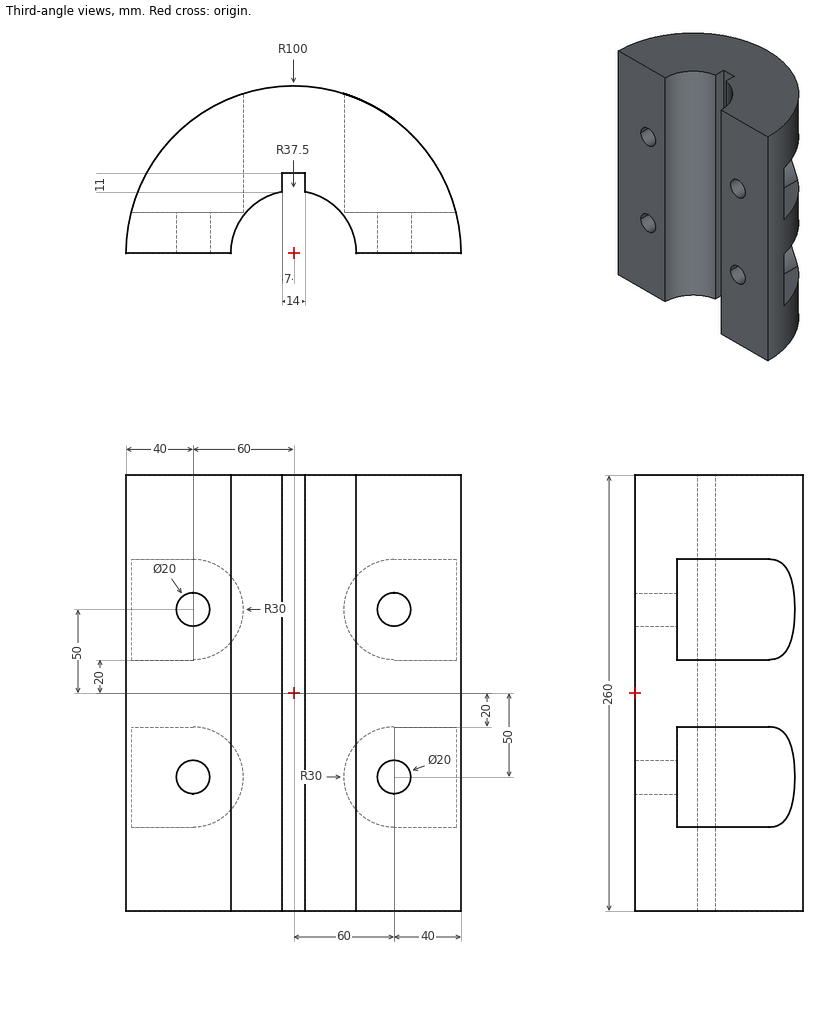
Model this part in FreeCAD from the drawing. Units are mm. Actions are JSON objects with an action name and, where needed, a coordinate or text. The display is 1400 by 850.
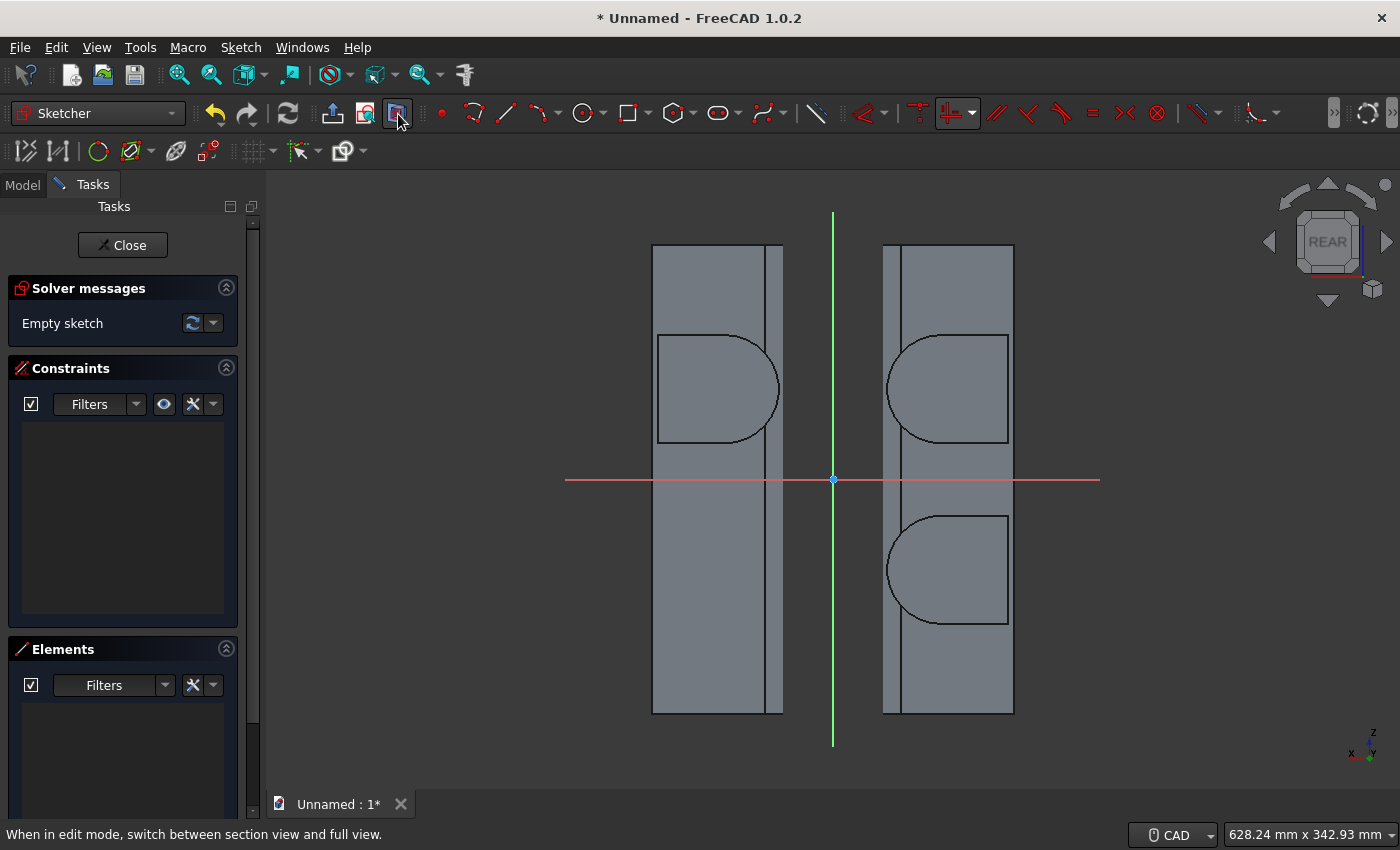
{"action": "scroll", "coordinate": [730, 594], "scroll_direction": "up", "scroll_amount": 5}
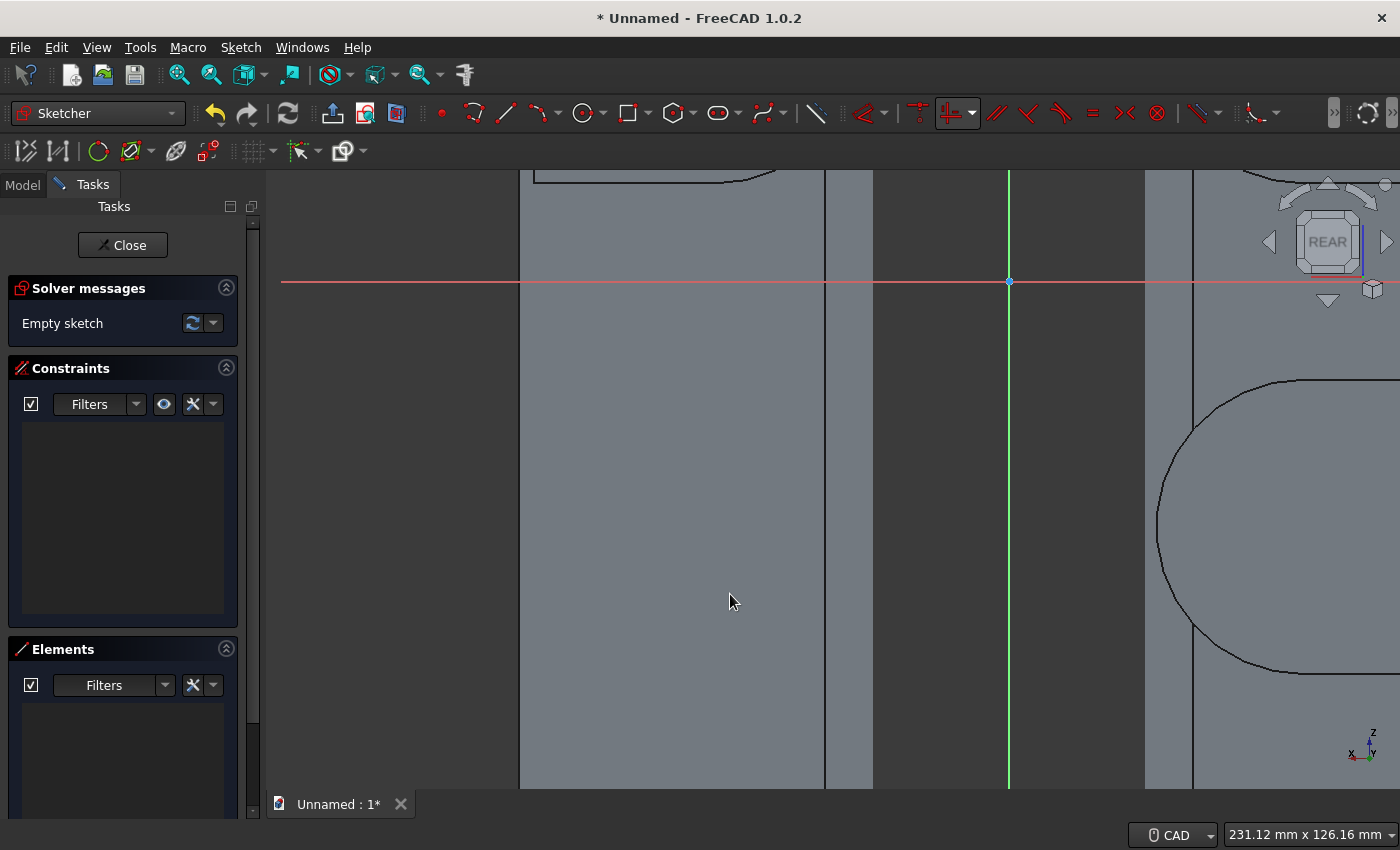
{"action": "left_click", "coordinate": [474, 114]}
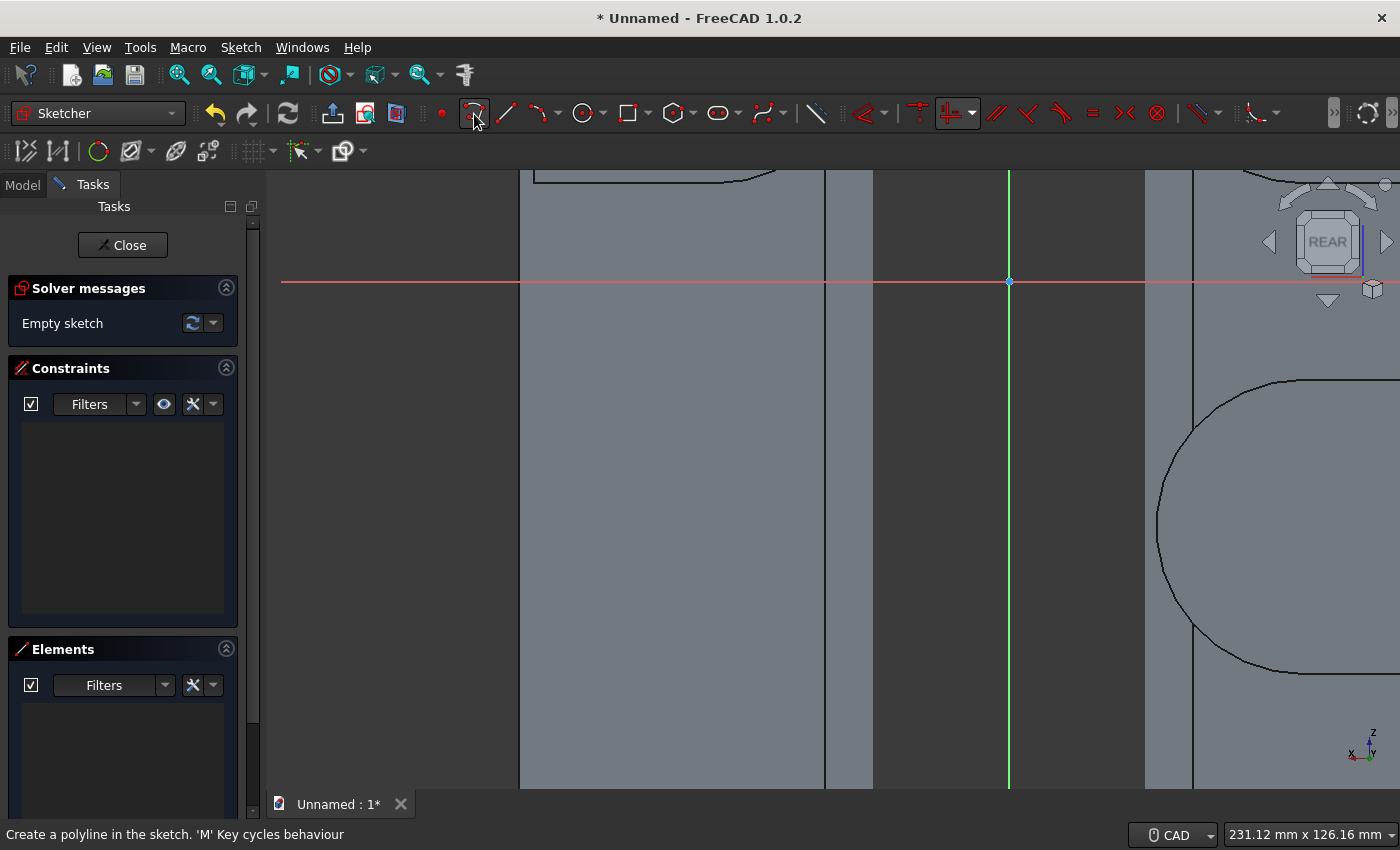
{"action": "left_click", "coordinate": [715, 380]}
{"action": "left_click", "coordinate": [519, 380]}
{"action": "left_click", "coordinate": [519, 674]}
{"action": "left_click", "coordinate": [715, 674]}
{"action": "right_click", "coordinate": [715, 674]}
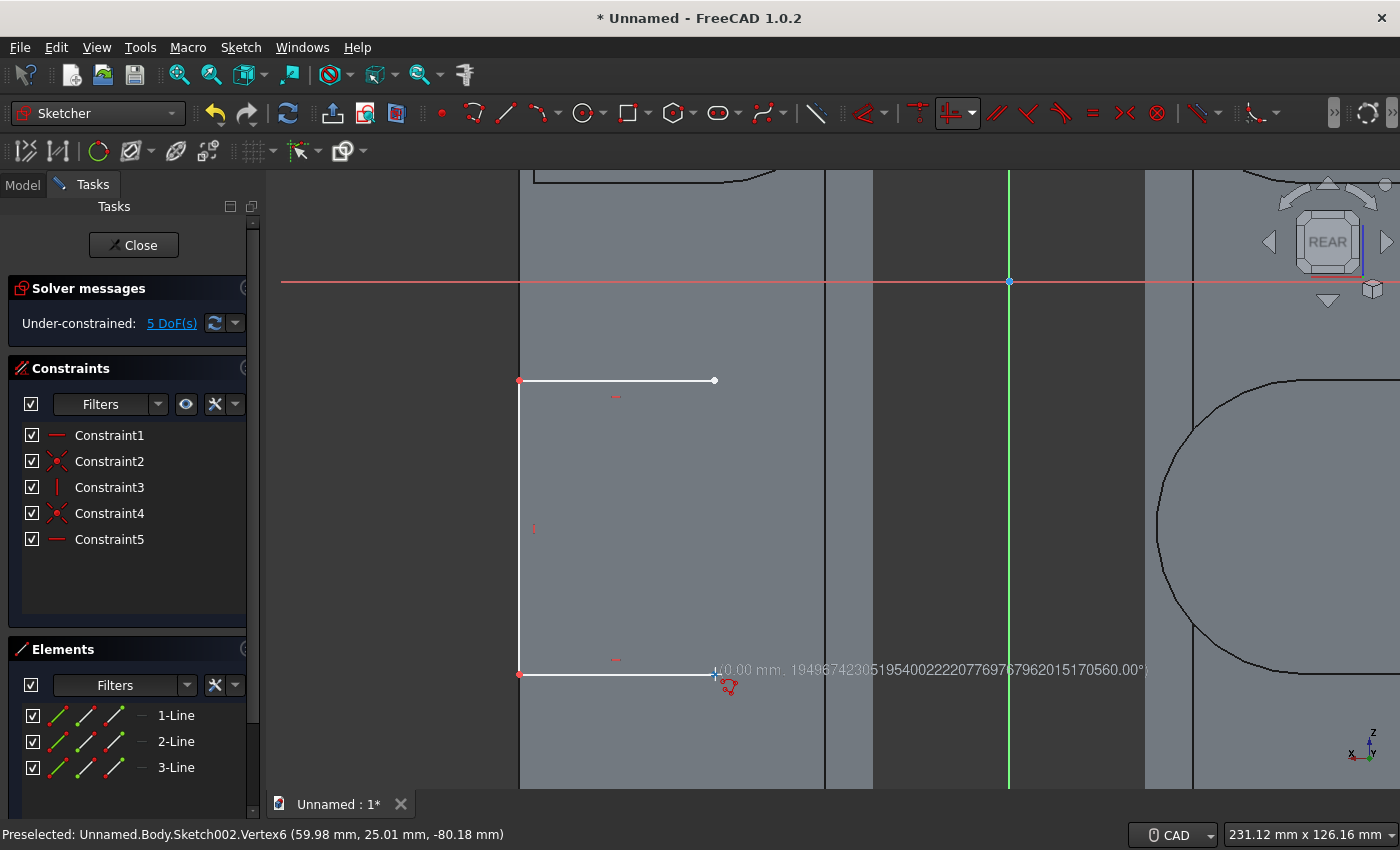
{"action": "left_click", "coordinate": [538, 114]}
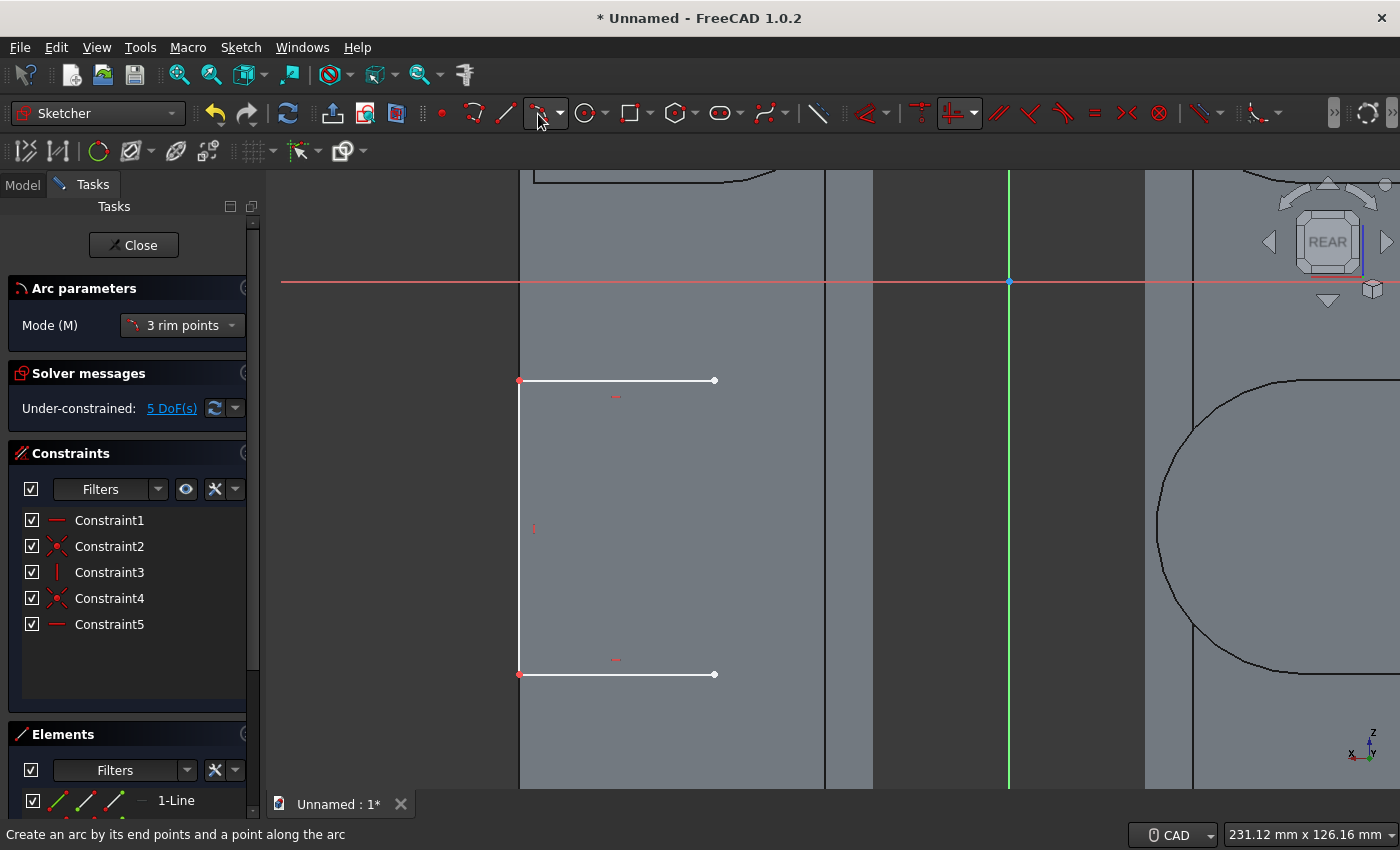
{"action": "left_click", "coordinate": [715, 675]}
{"action": "left_click", "coordinate": [715, 381]}
{"action": "left_click", "coordinate": [862, 527]}
{"action": "key", "text": "Escape"}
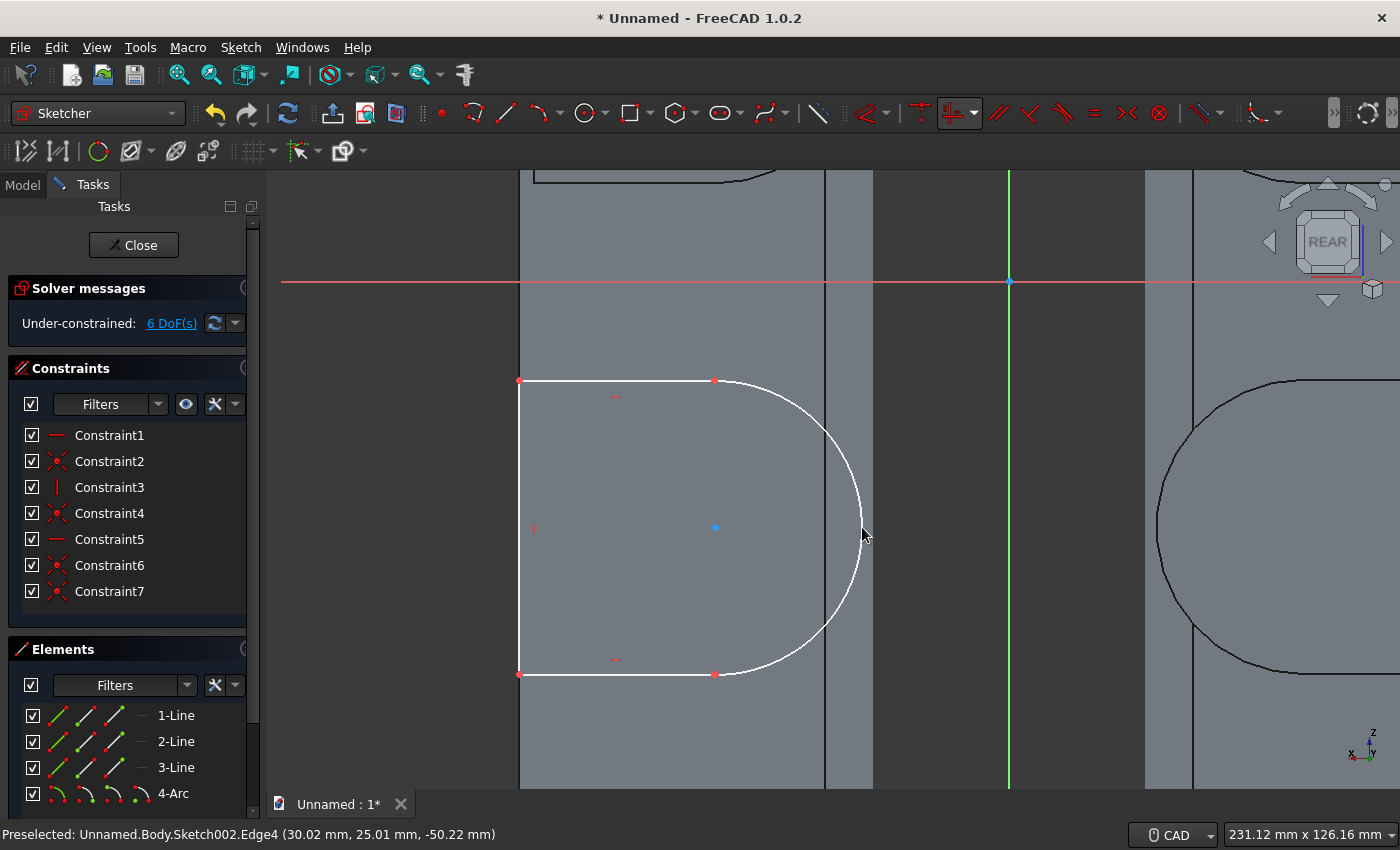
{"action": "left_click", "coordinate": [656, 381]}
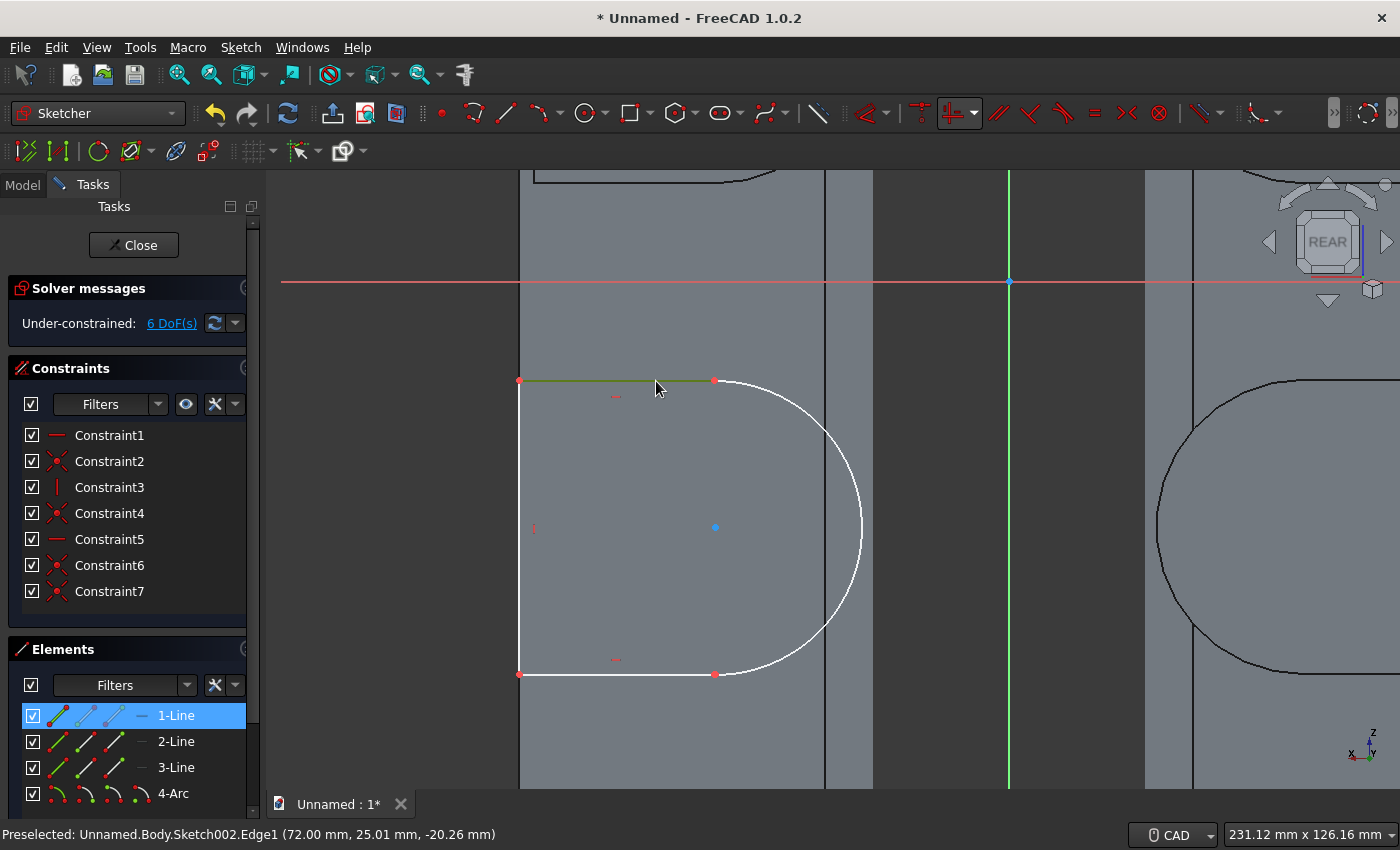
{"action": "left_click", "coordinate": [834, 614]}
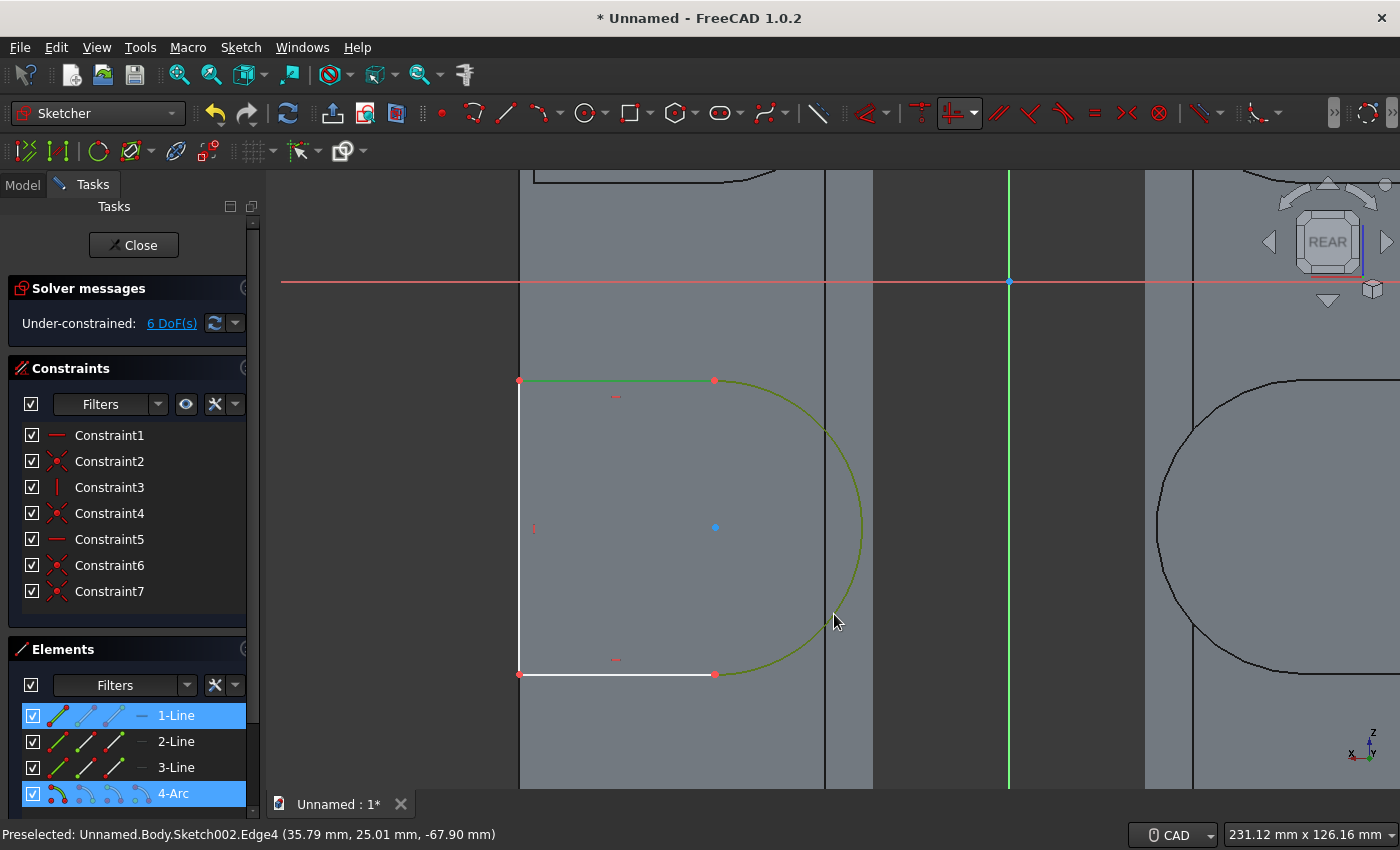
{"action": "left_click", "coordinate": [1064, 114]}